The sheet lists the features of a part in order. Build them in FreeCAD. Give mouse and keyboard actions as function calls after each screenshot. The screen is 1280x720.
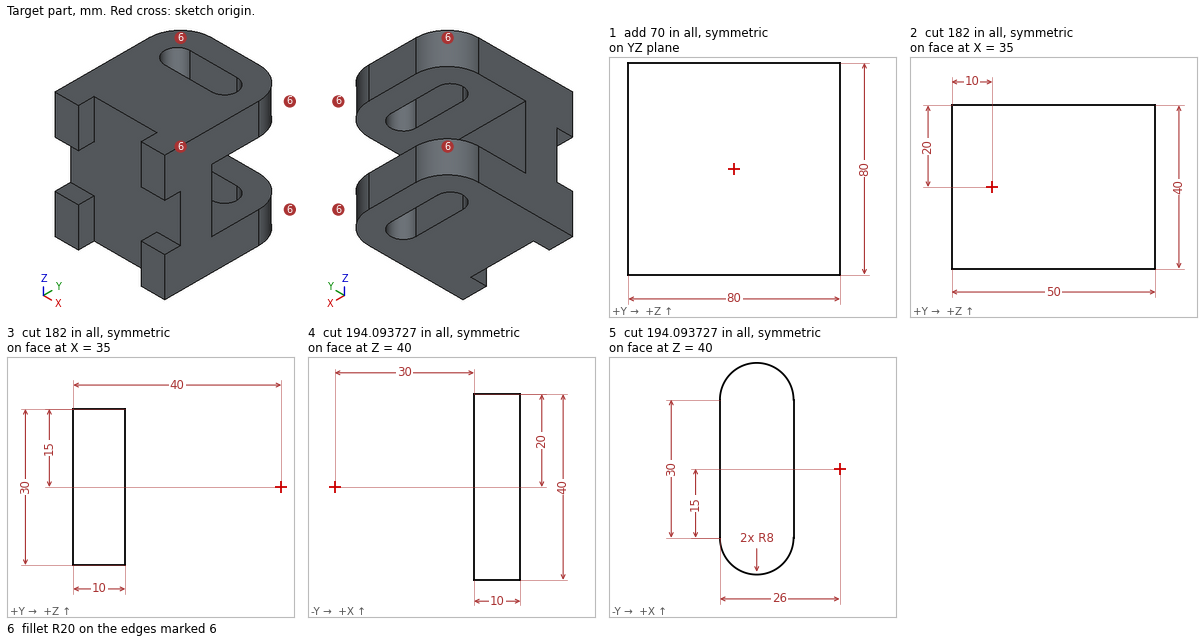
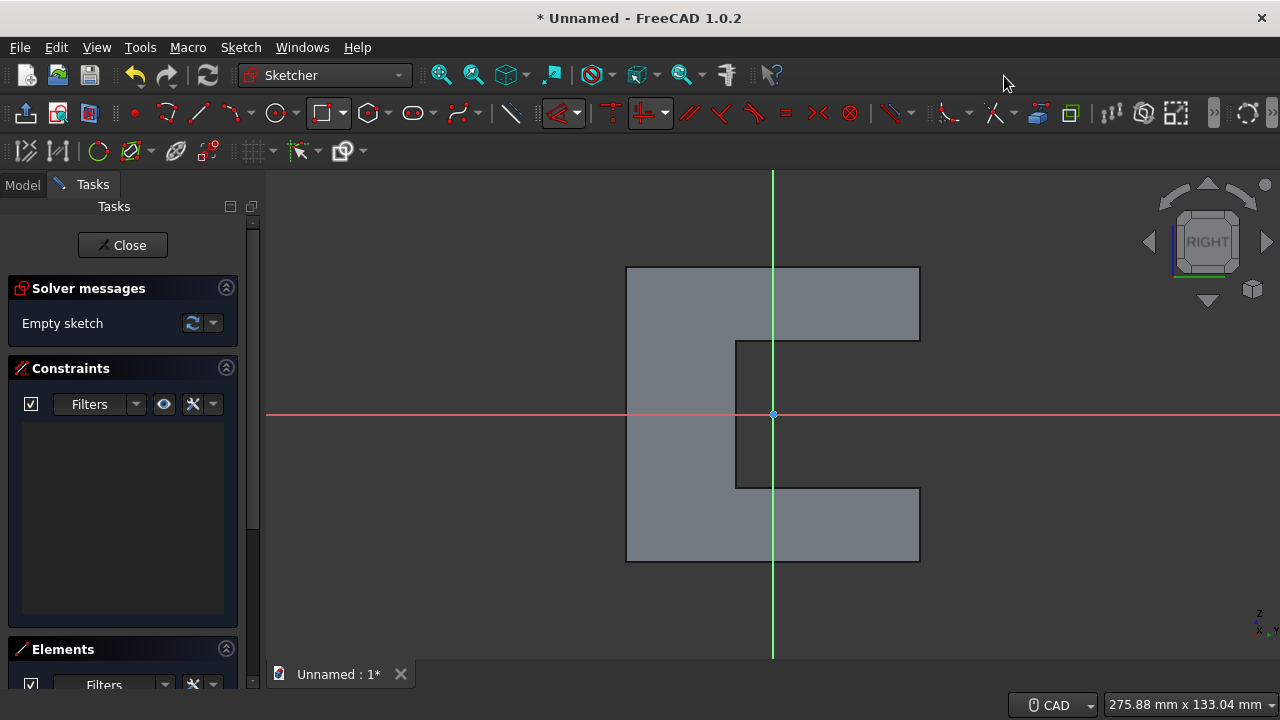
scroll(697, 414, up, 5)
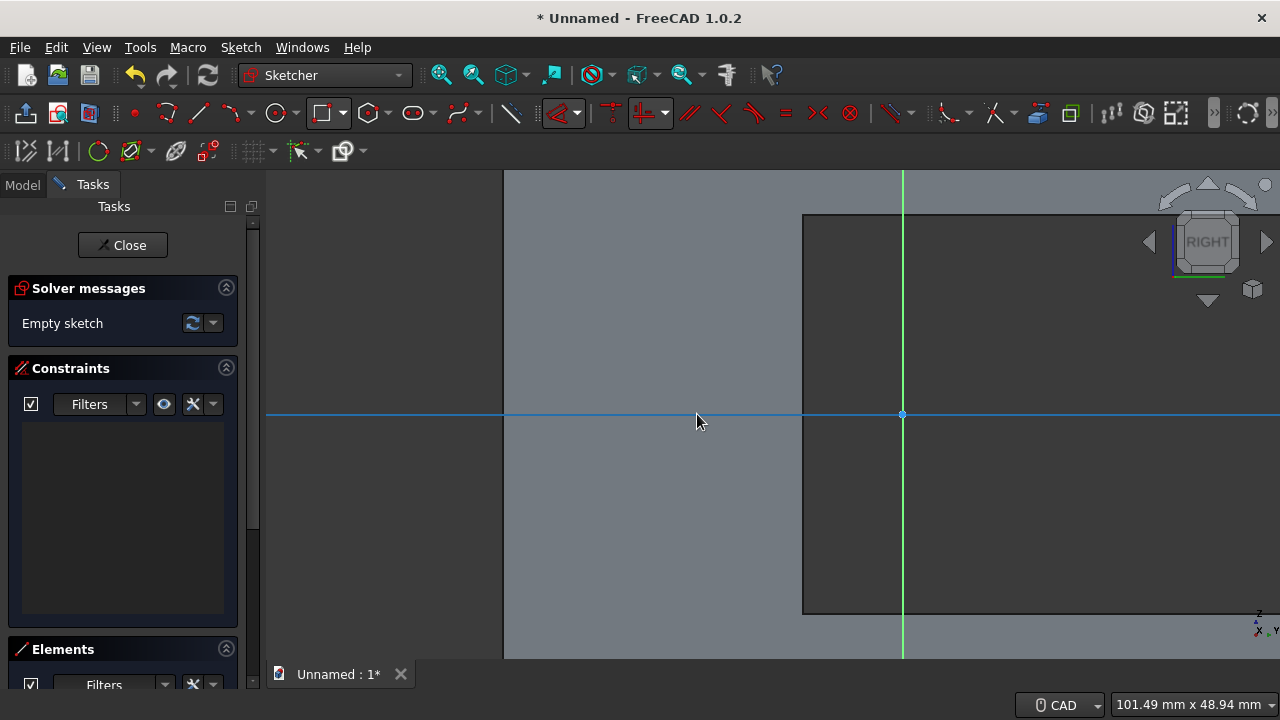
key(g)
key(r)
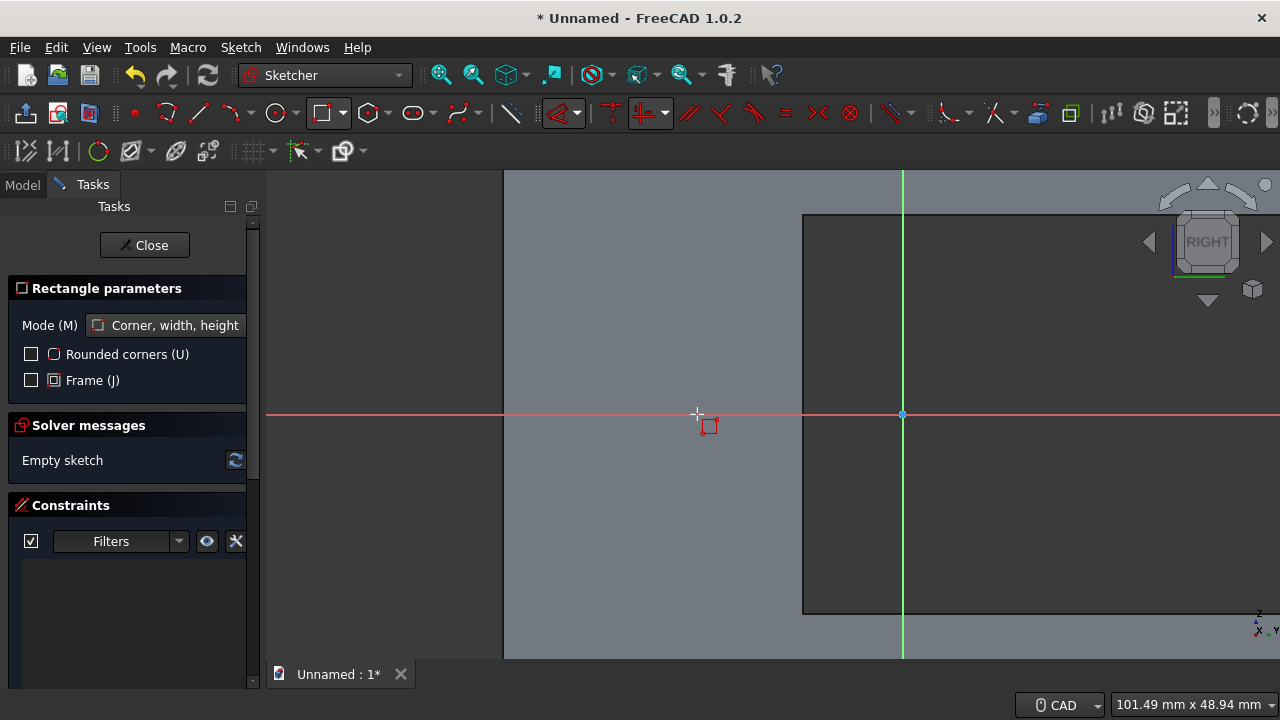
click(503, 265)
move(603, 564)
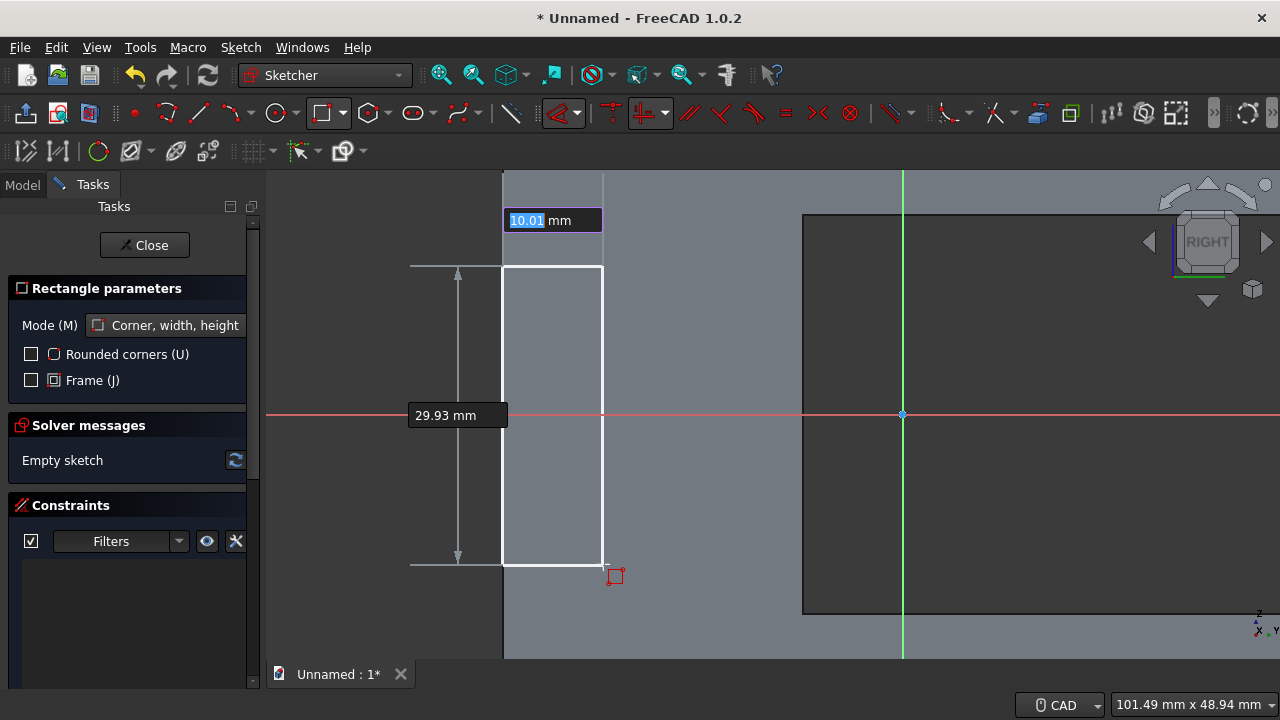
text(10)
key(Tab)
text(30)
key(Return)
key(Escape)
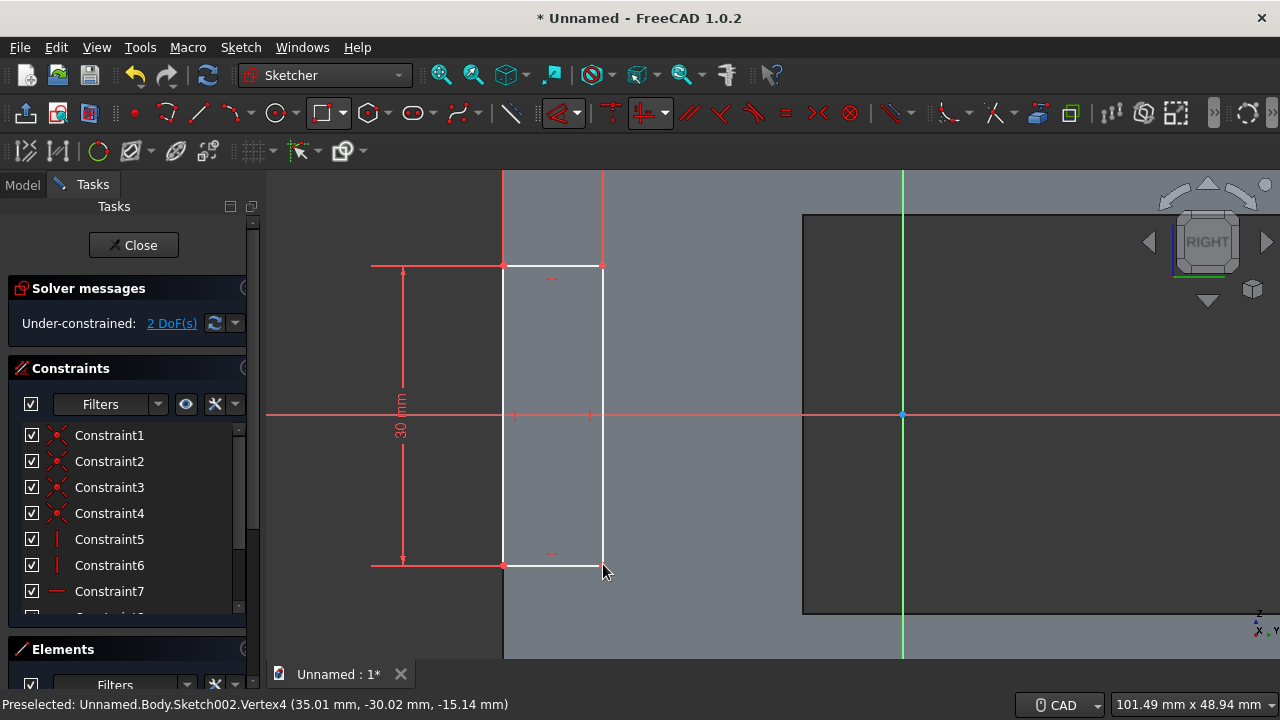
click(558, 114)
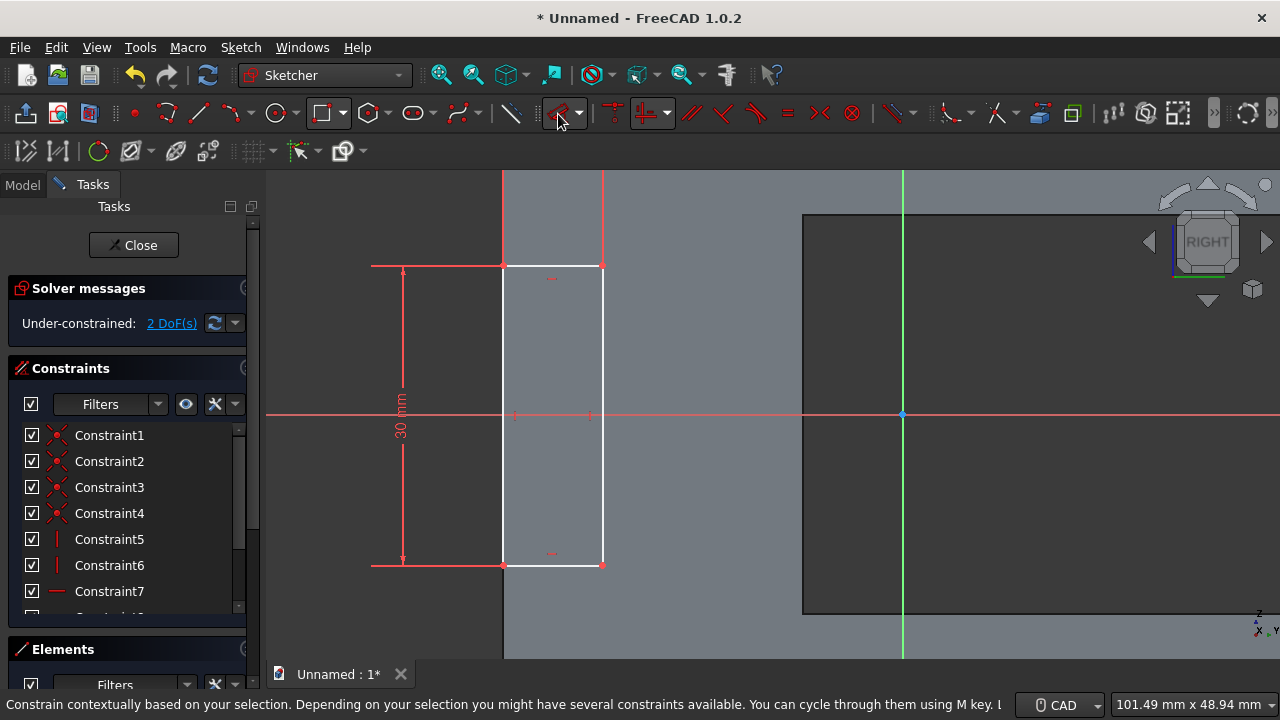
click(503, 266)
click(703, 232)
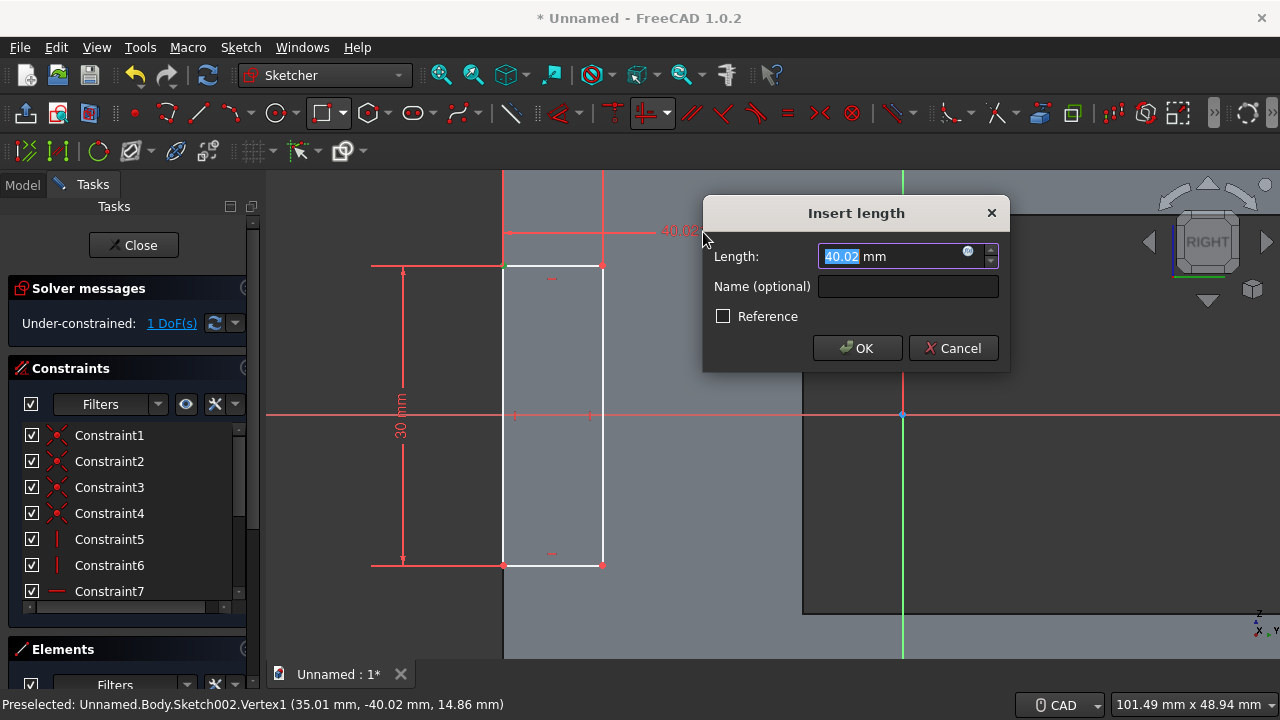
text(40)
key(Return)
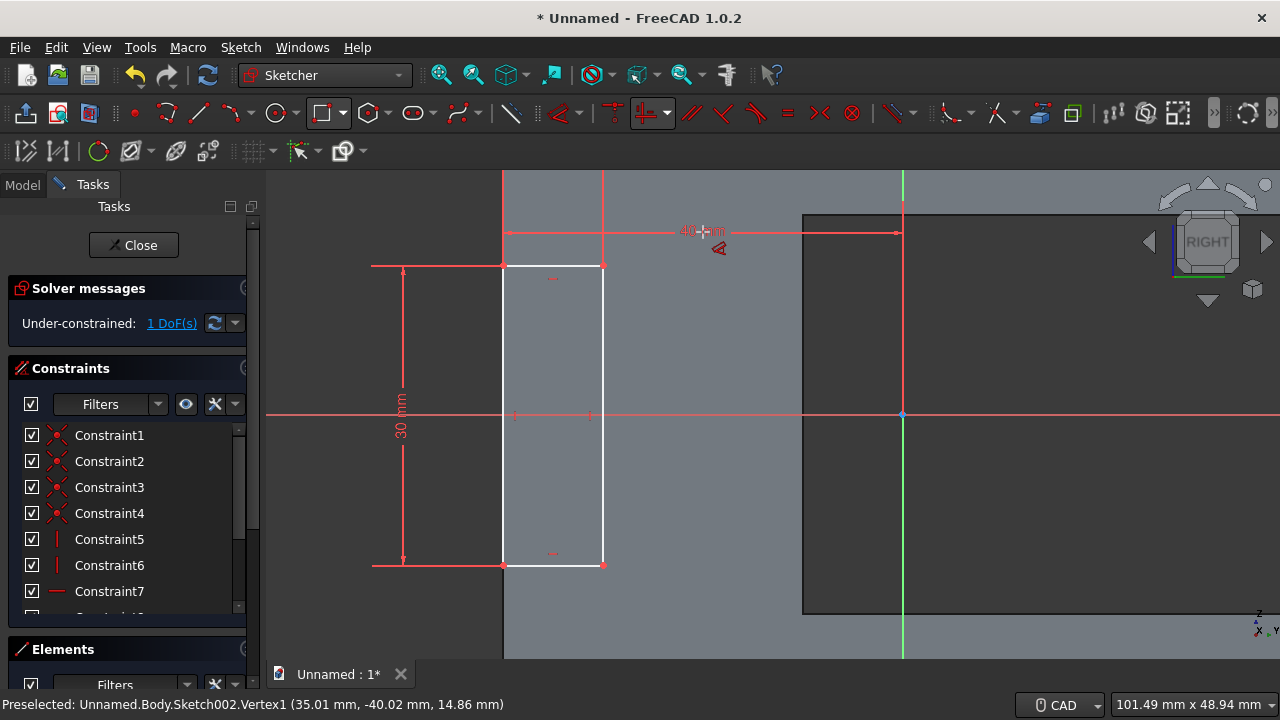
click(503, 266)
click(937, 340)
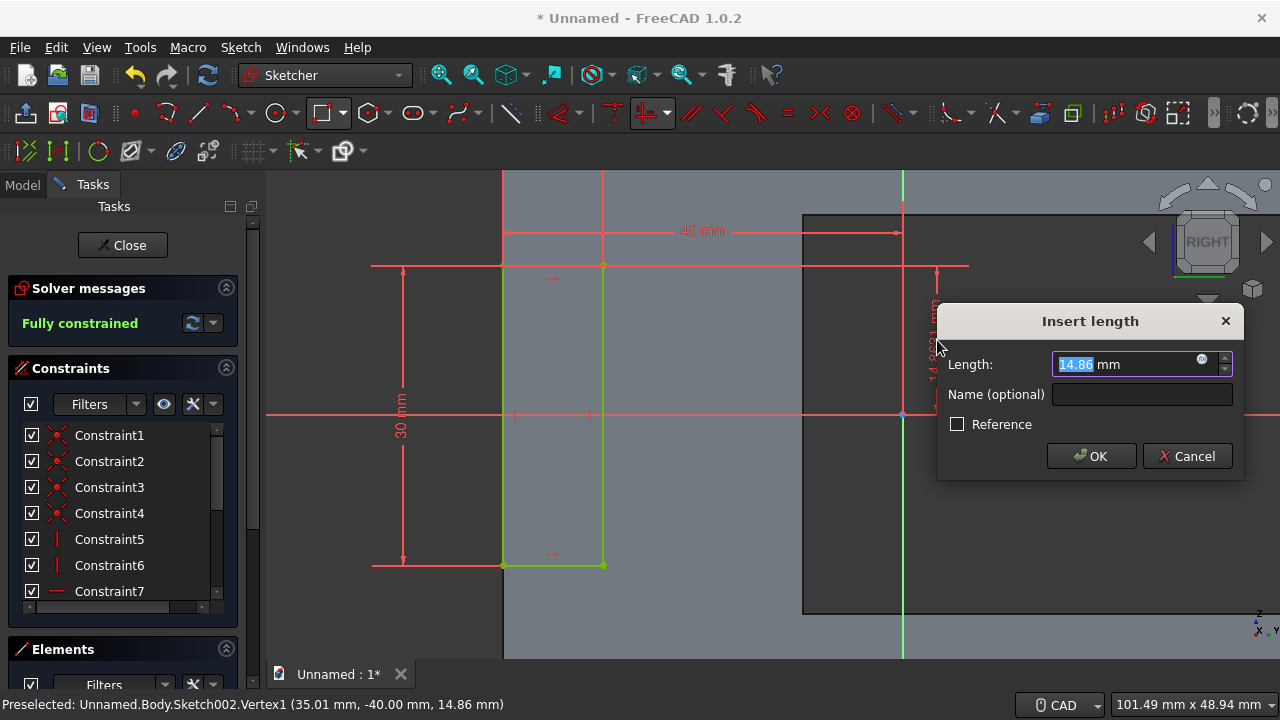
text(15)
key(Return)
key(Escape)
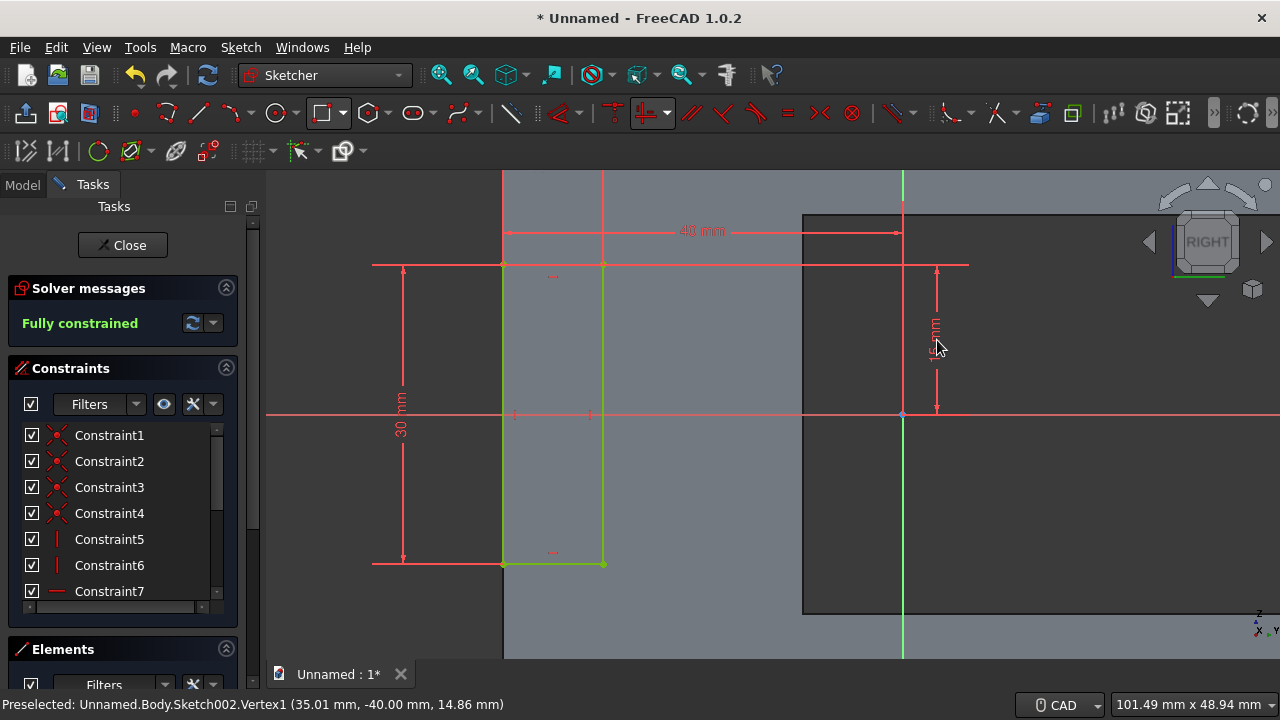
click(123, 245)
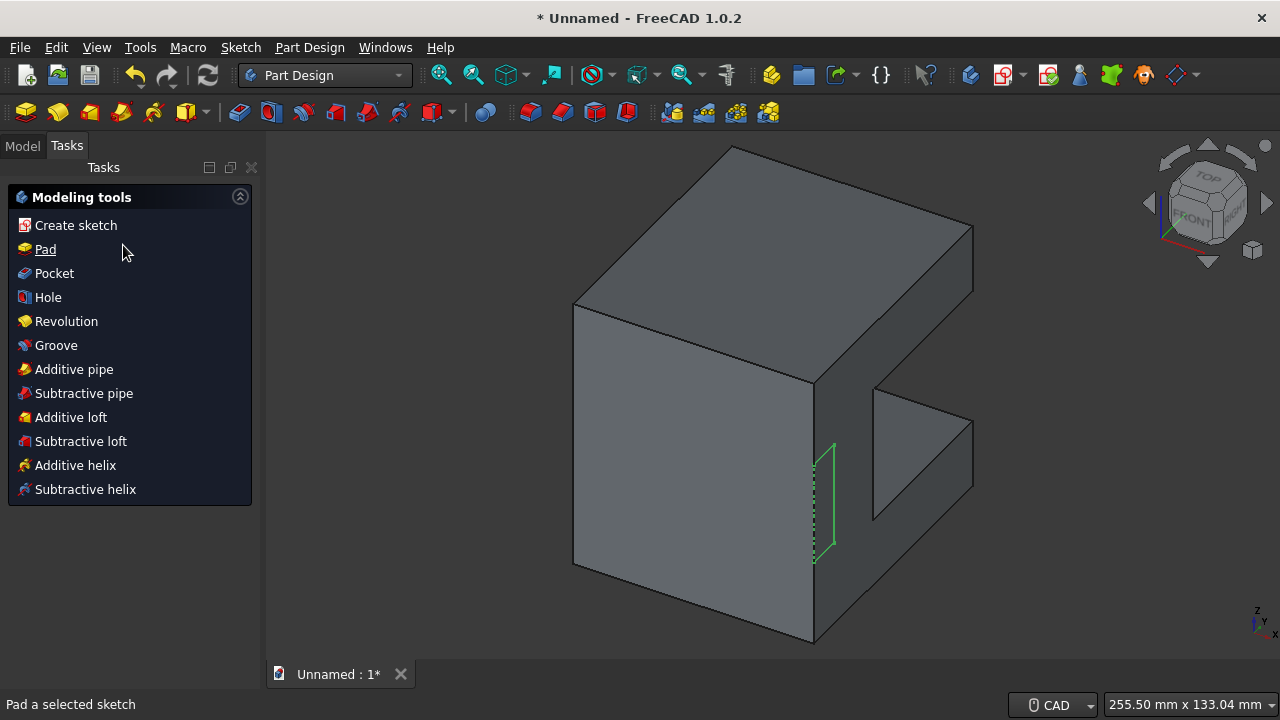
click(240, 112)